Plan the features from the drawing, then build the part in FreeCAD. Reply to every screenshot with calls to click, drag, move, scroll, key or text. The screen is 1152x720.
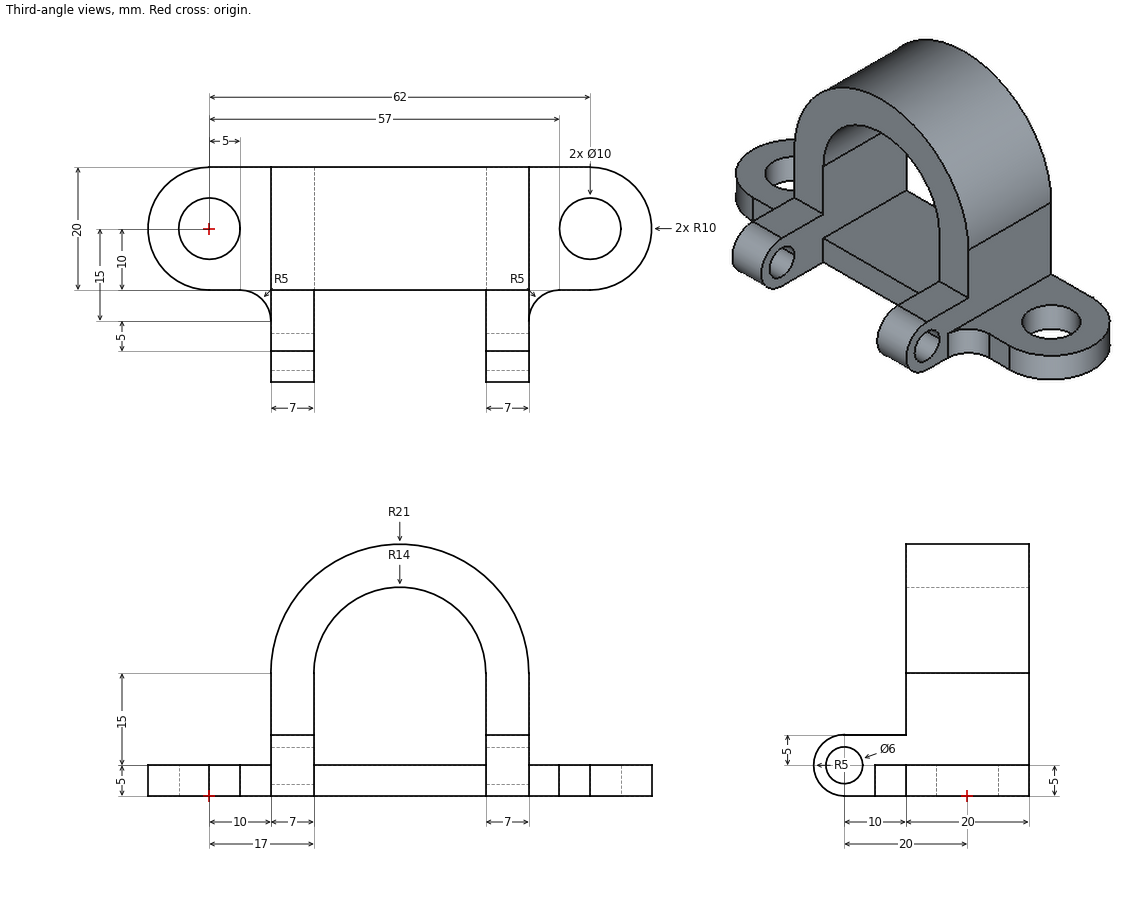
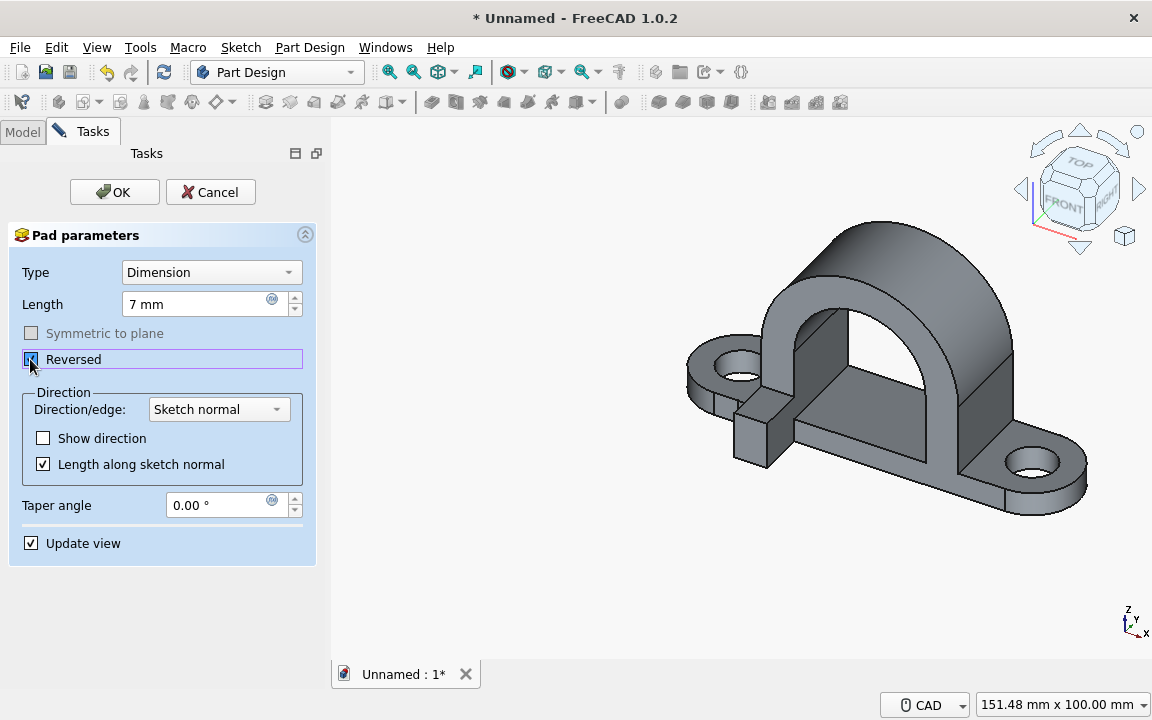
click(115, 192)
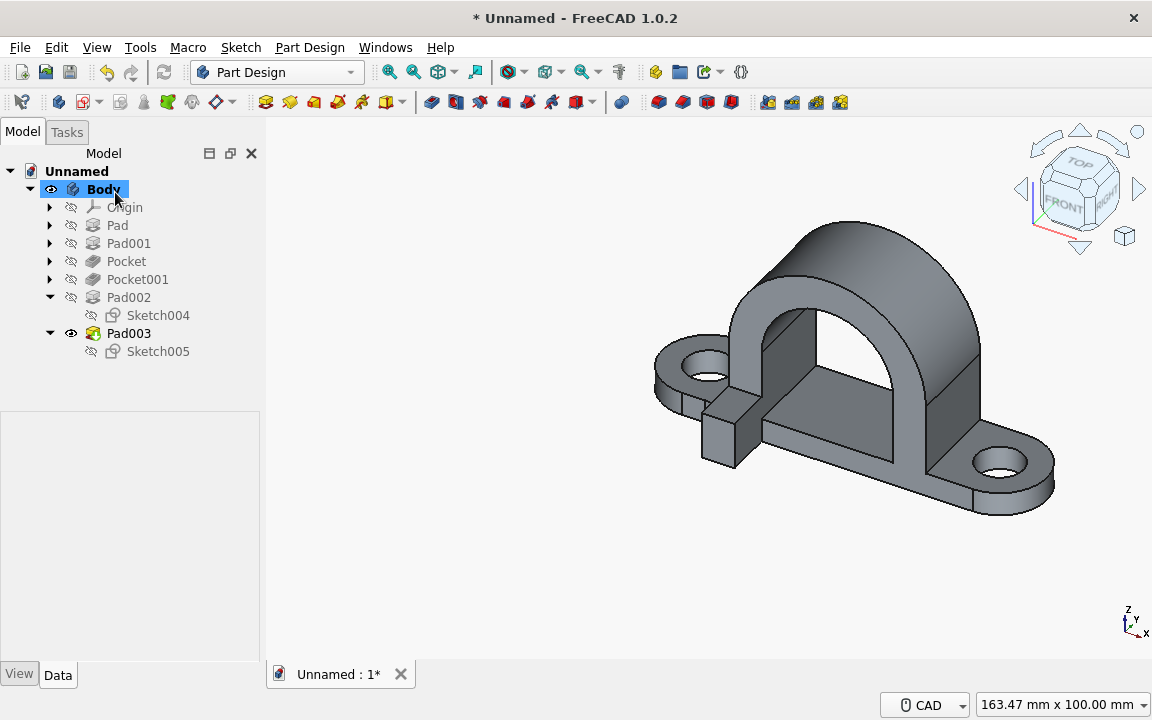
click(679, 377)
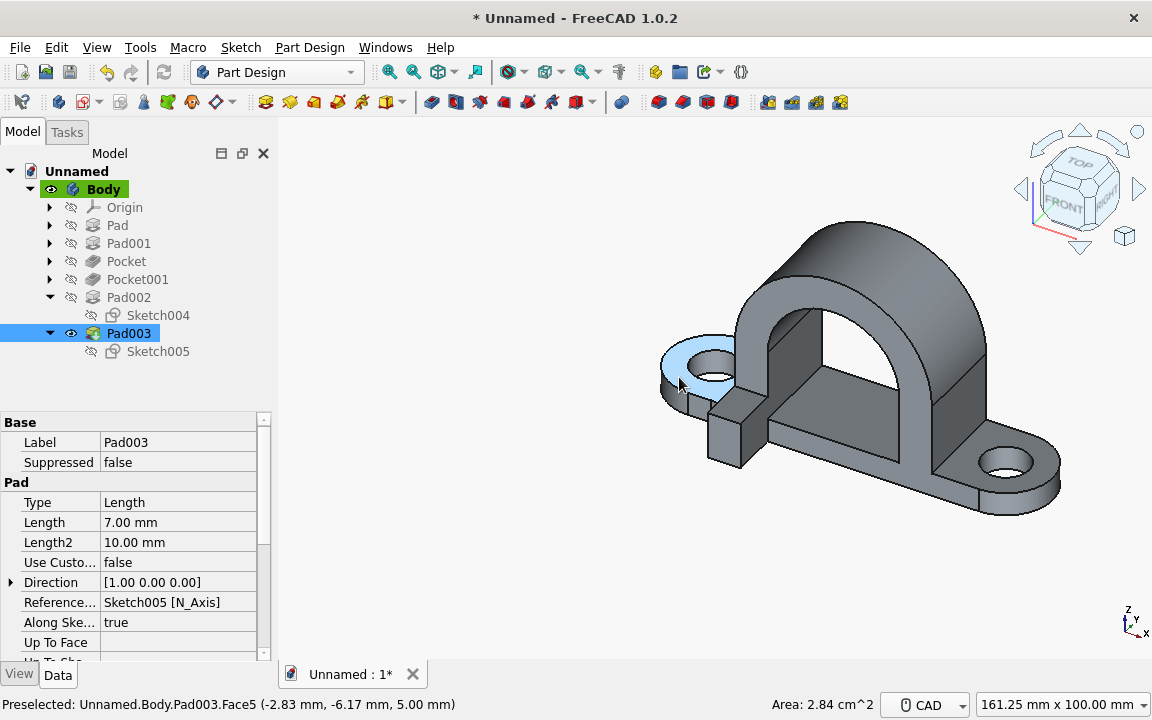
click(84, 102)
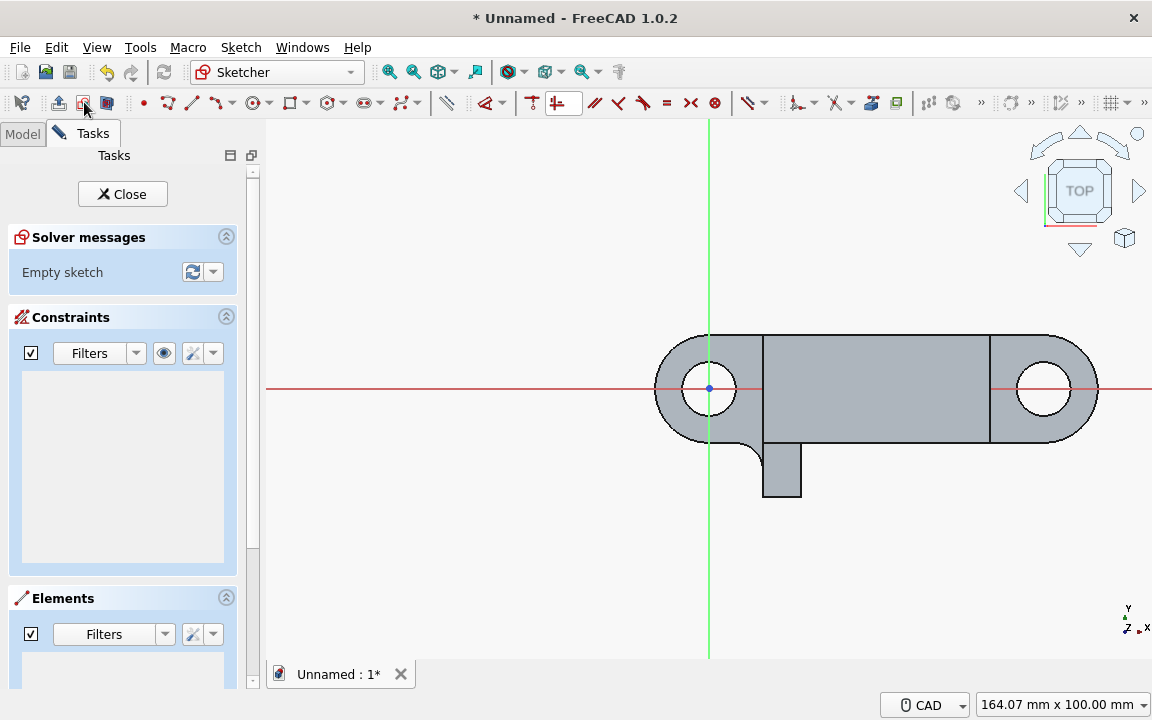
key(q)
key(s)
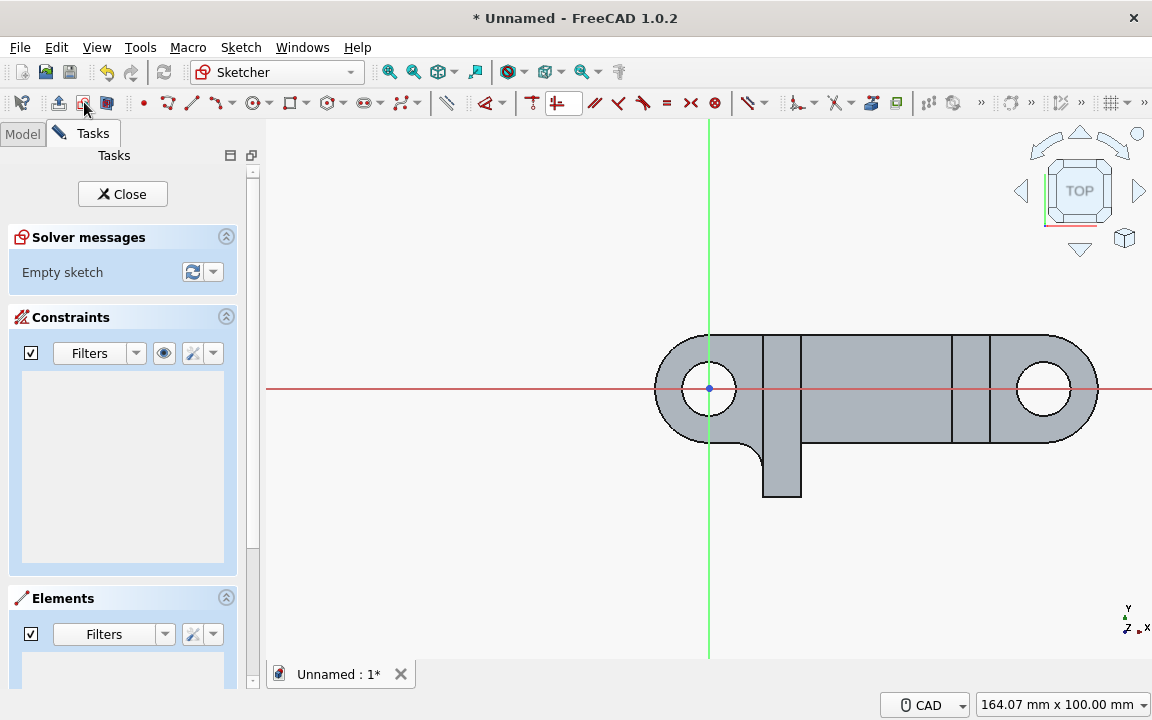
scroll(640, 389, down, 5)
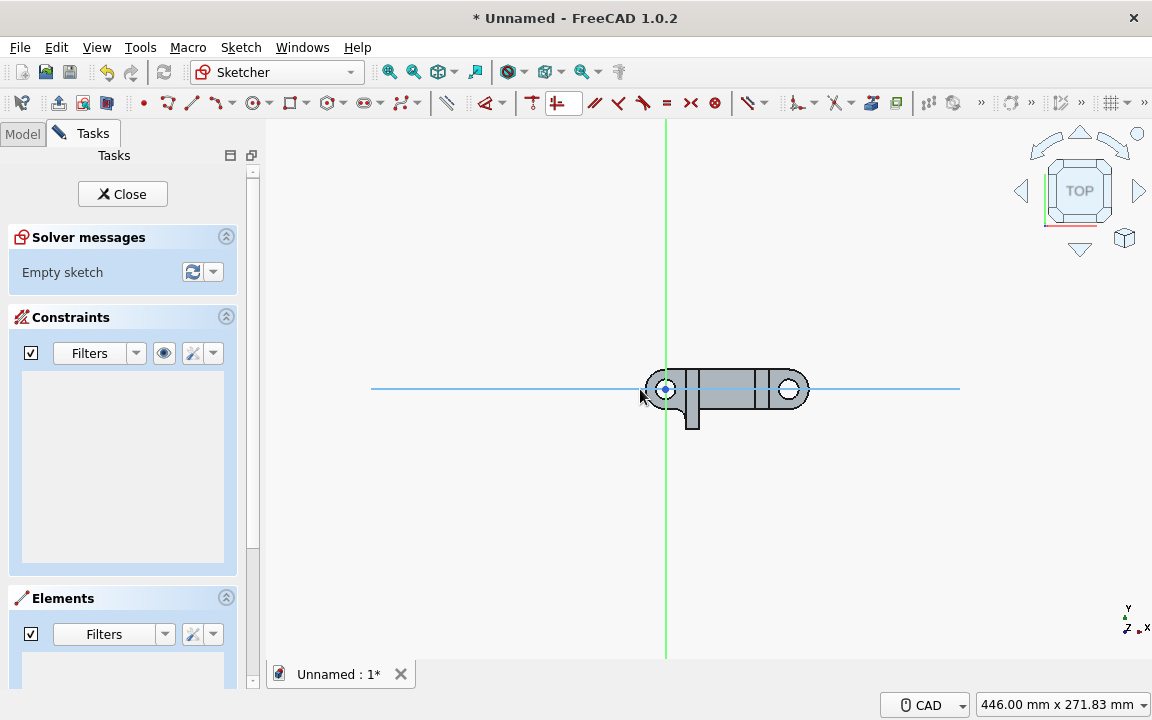
scroll(775, 421, up, 14)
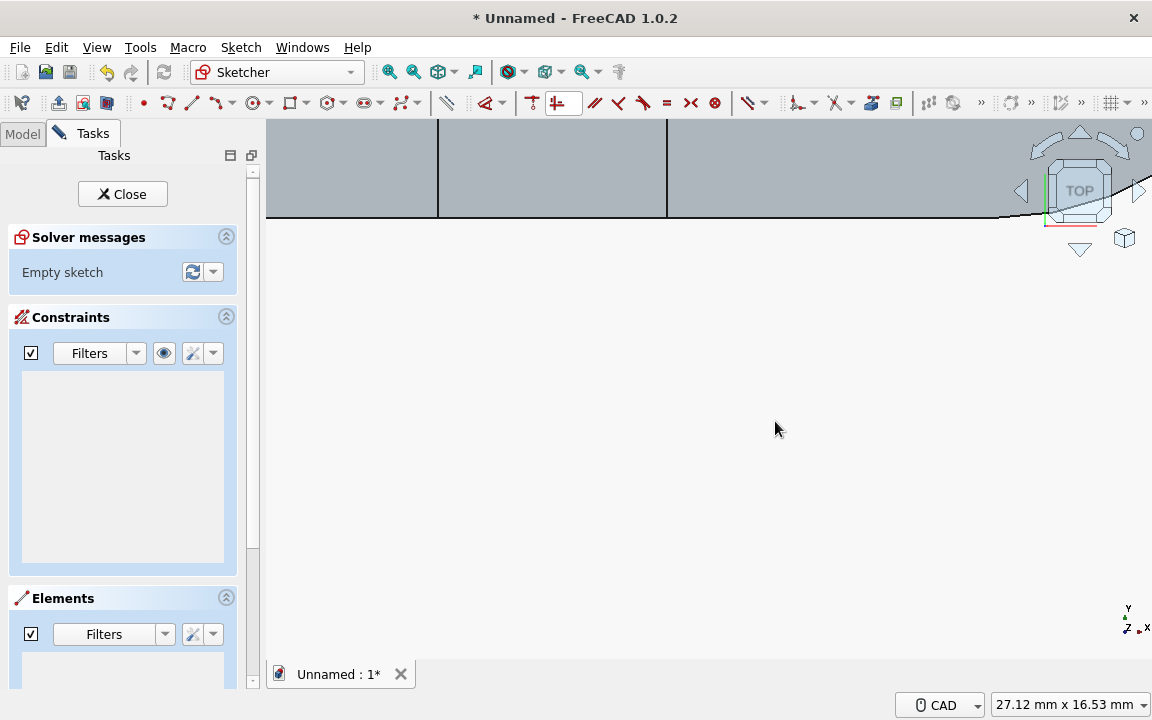
key(g)
key(m)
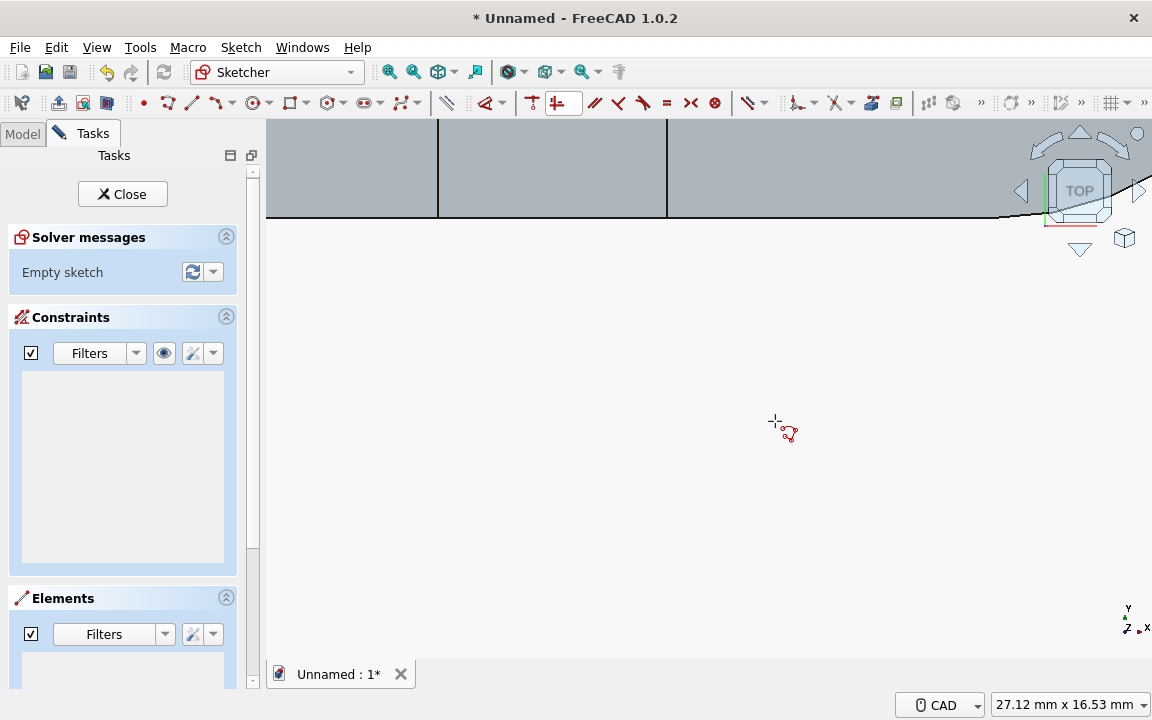
click(830, 218)
click(438, 218)
click(438, 545)
click(667, 545)
click(667, 381)
right_click(667, 381)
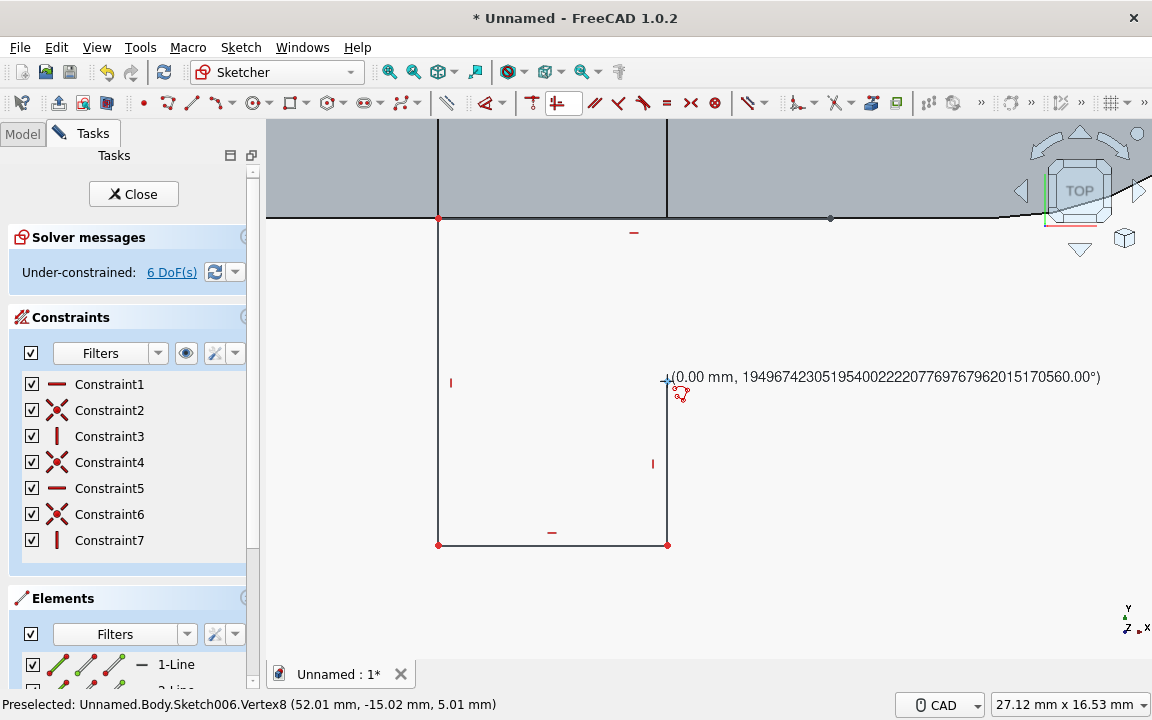
click(216, 104)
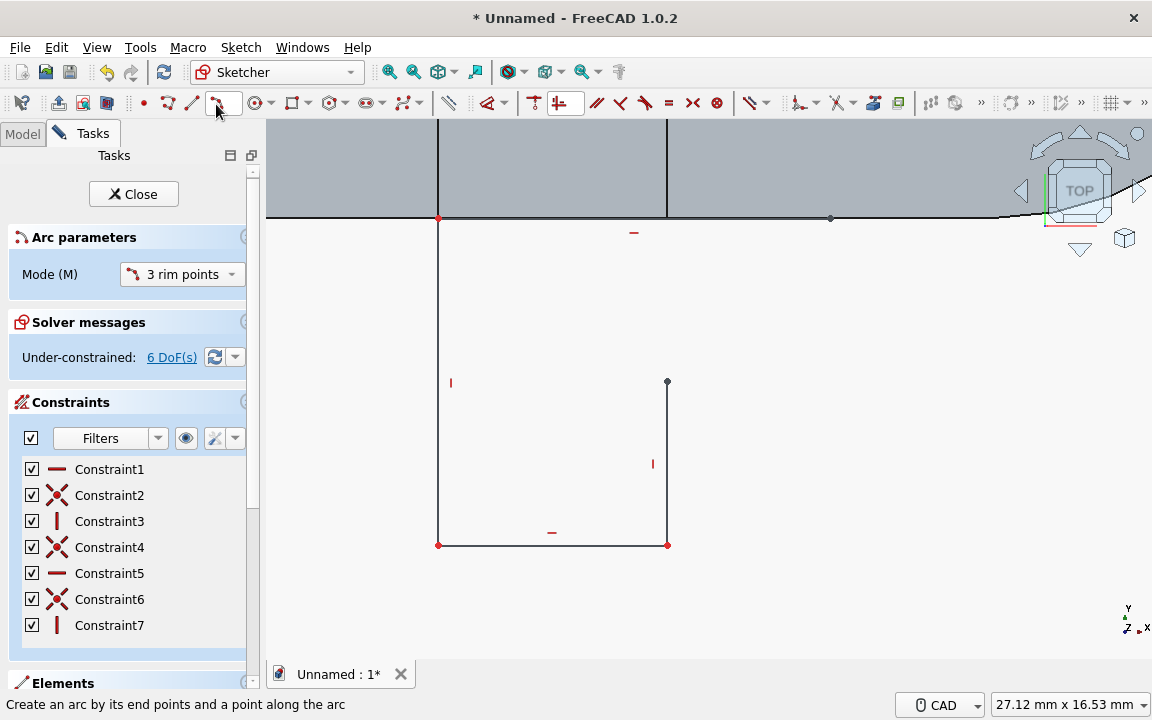
click(667, 382)
click(830, 219)
click(714, 266)
key(Escape)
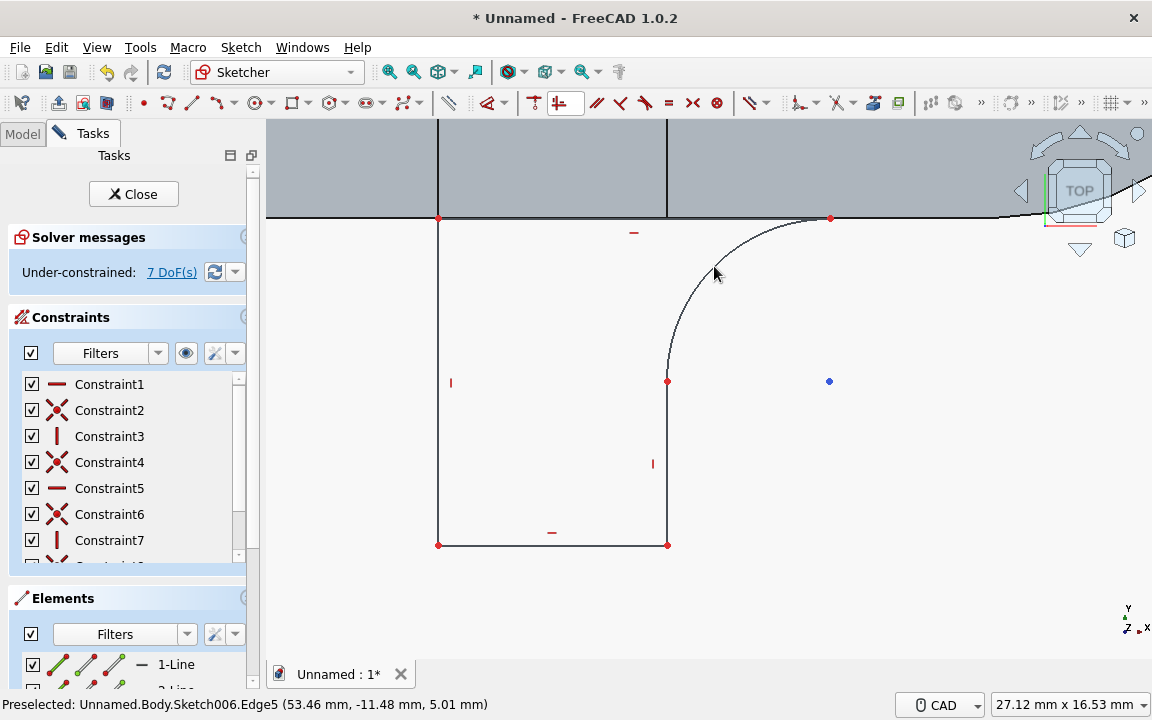
click(712, 219)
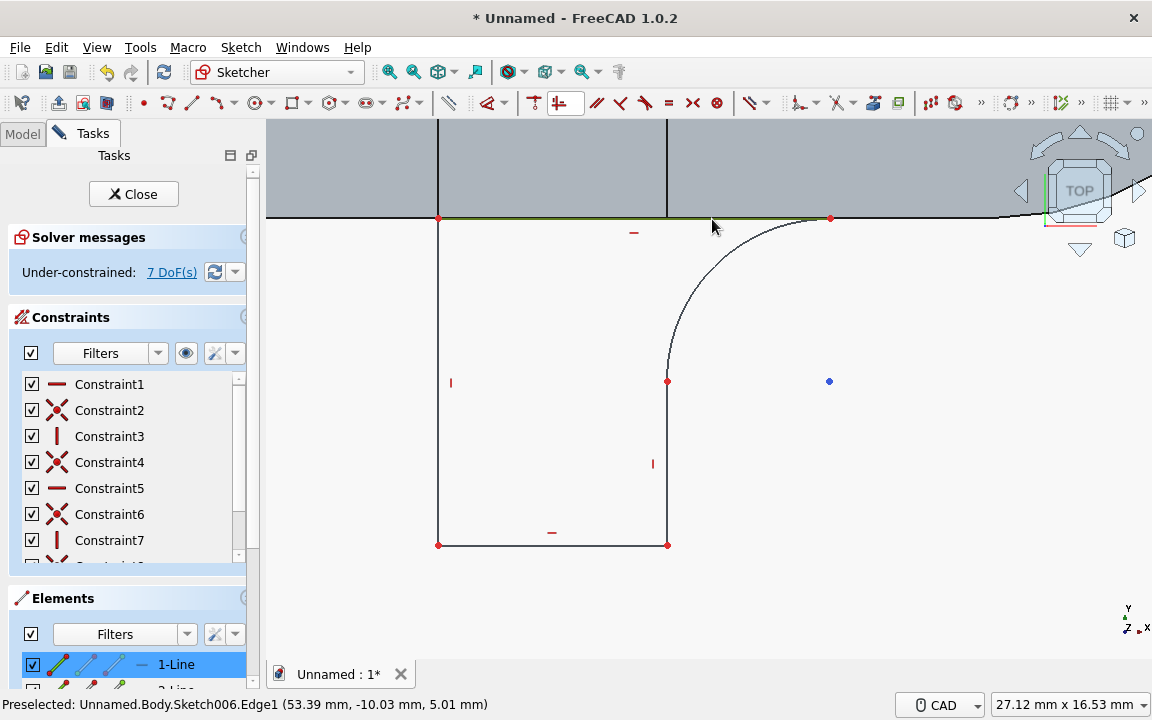
click(756, 237)